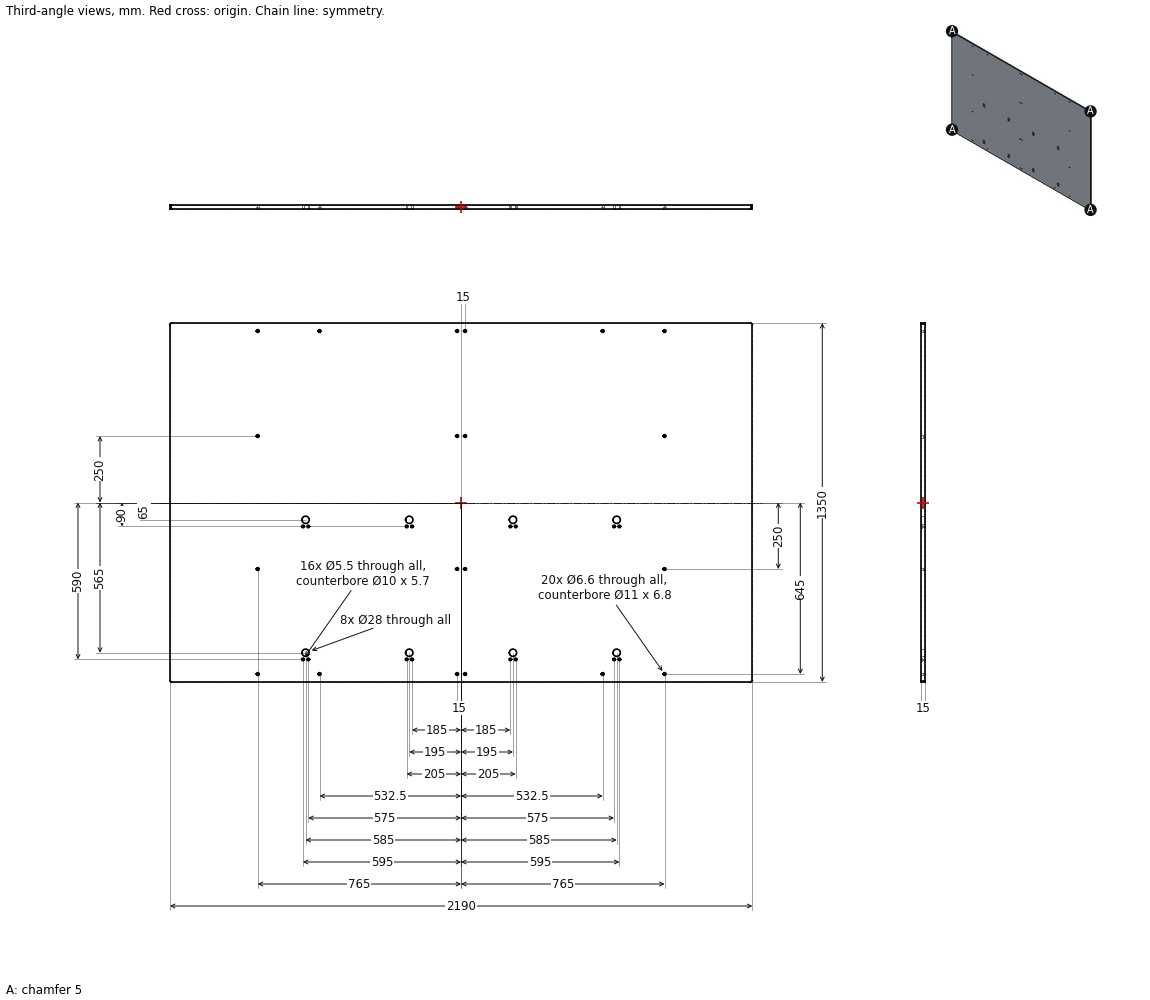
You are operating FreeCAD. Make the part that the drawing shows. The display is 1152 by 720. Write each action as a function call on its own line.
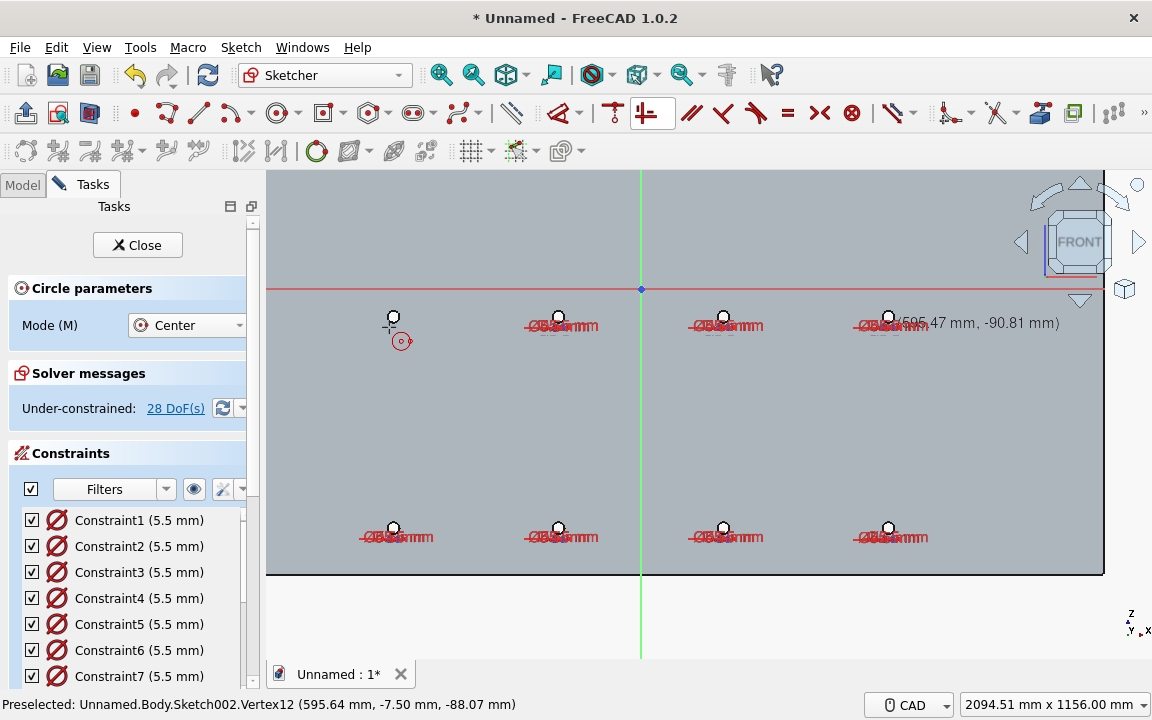
click(389, 327)
move(390, 326)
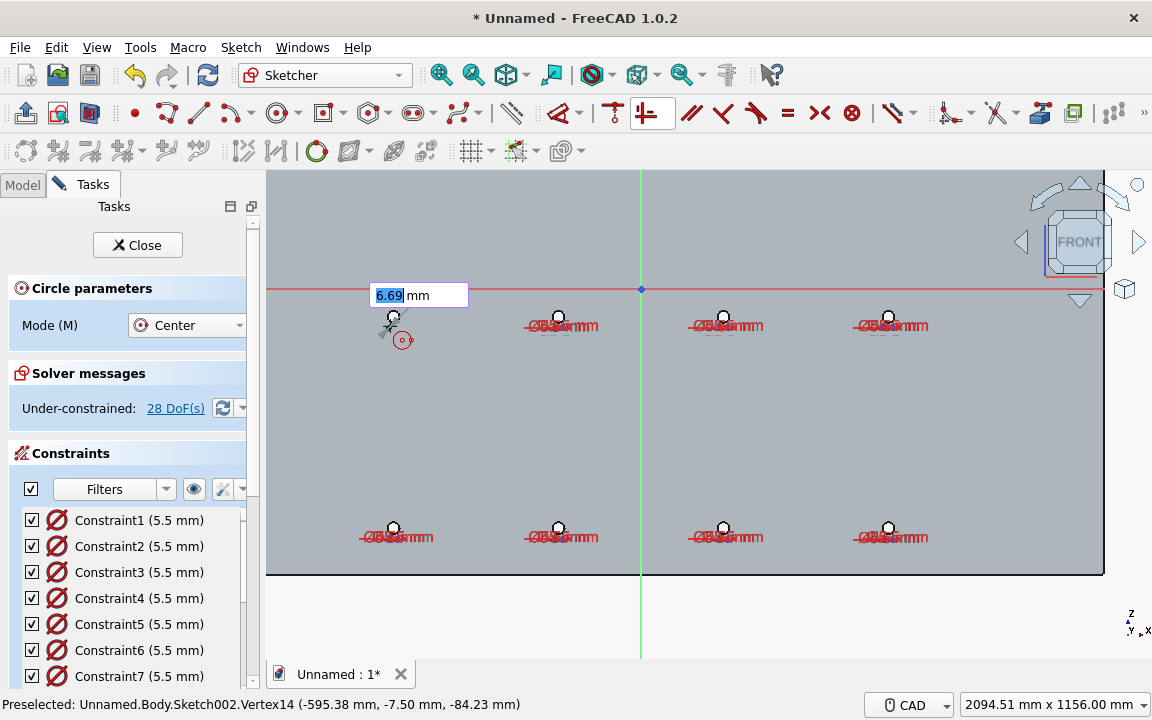
text(5.5)
key(Return)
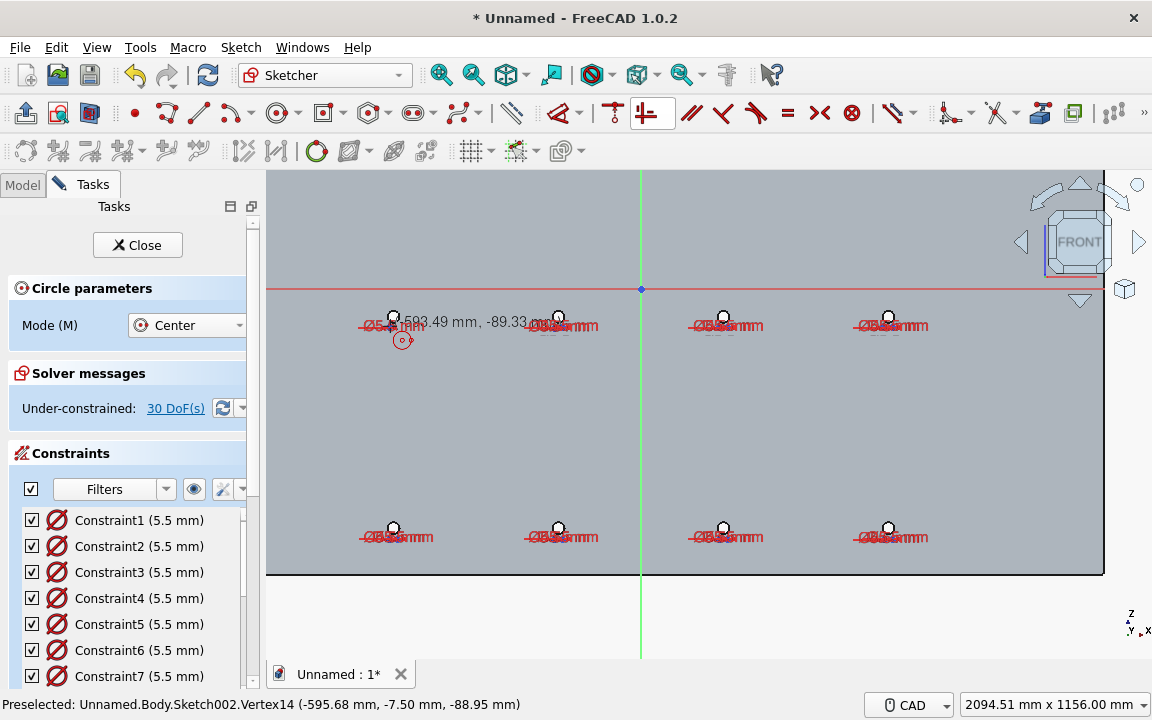
scroll(398, 327, up, 15)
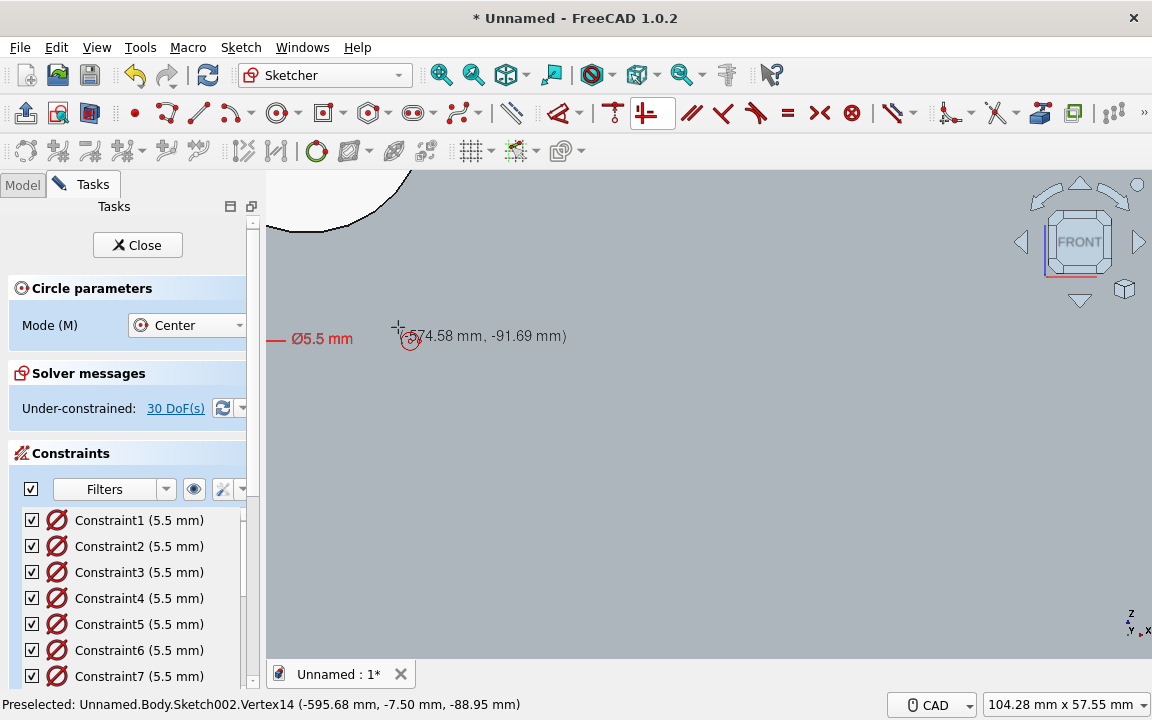
scroll(398, 327, down, 15)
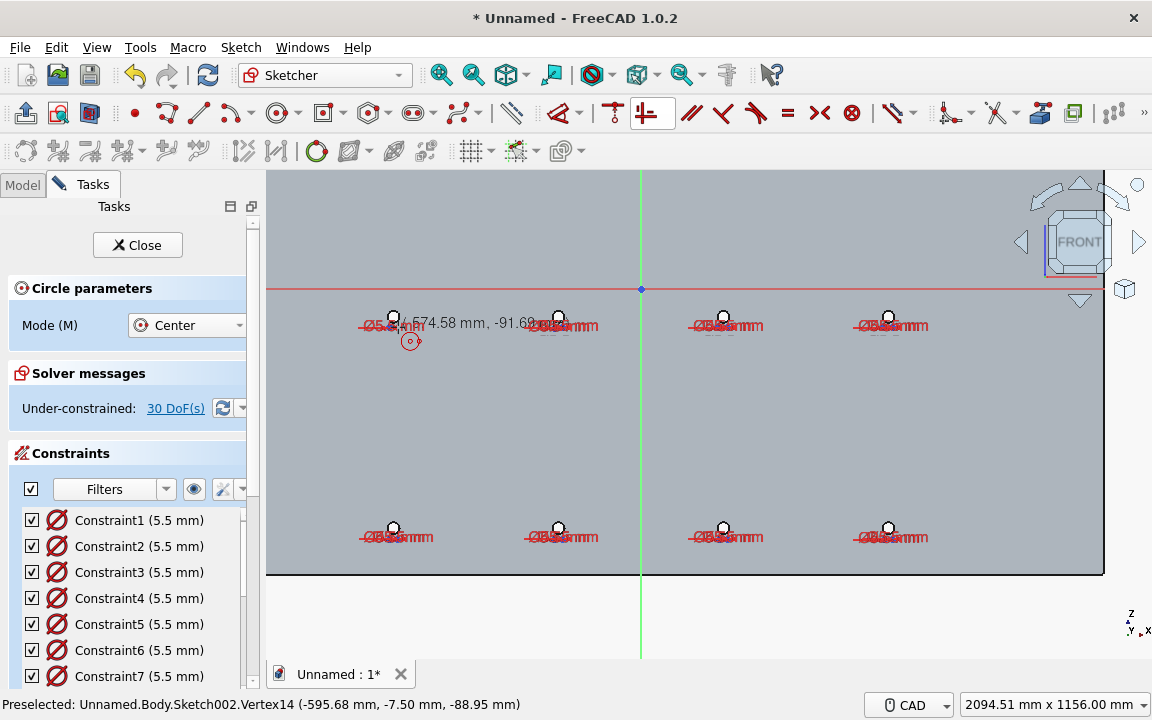
scroll(398, 327, up, 4)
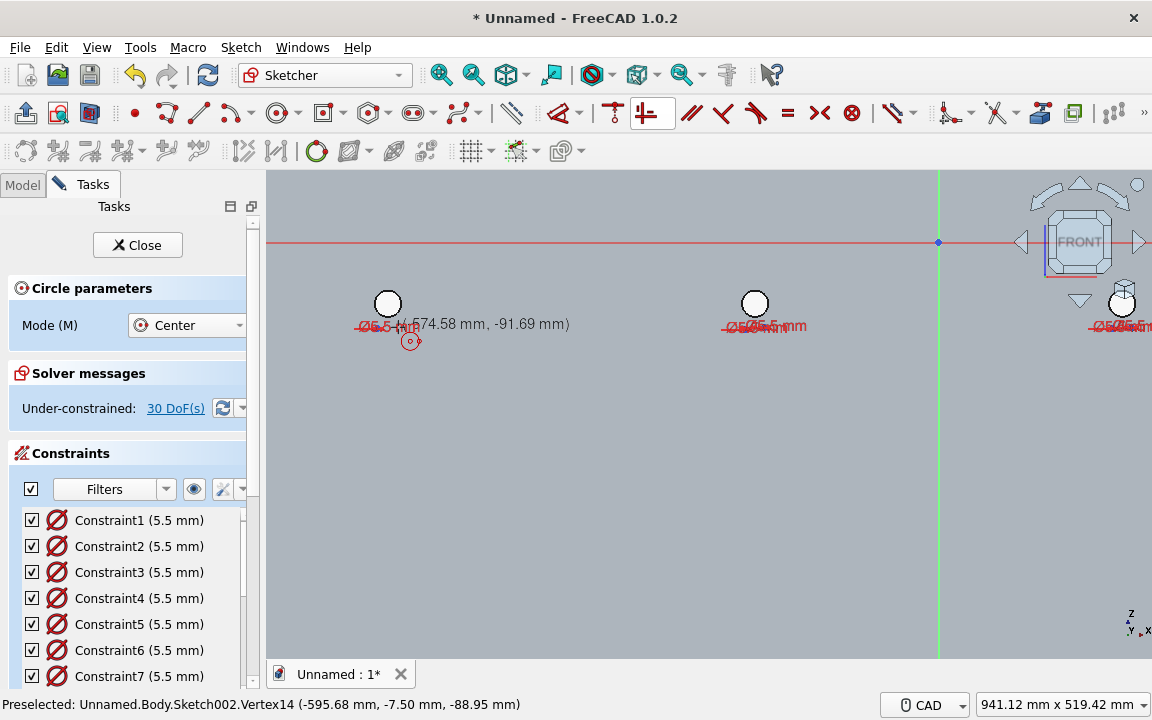
click(397, 327)
move(399, 325)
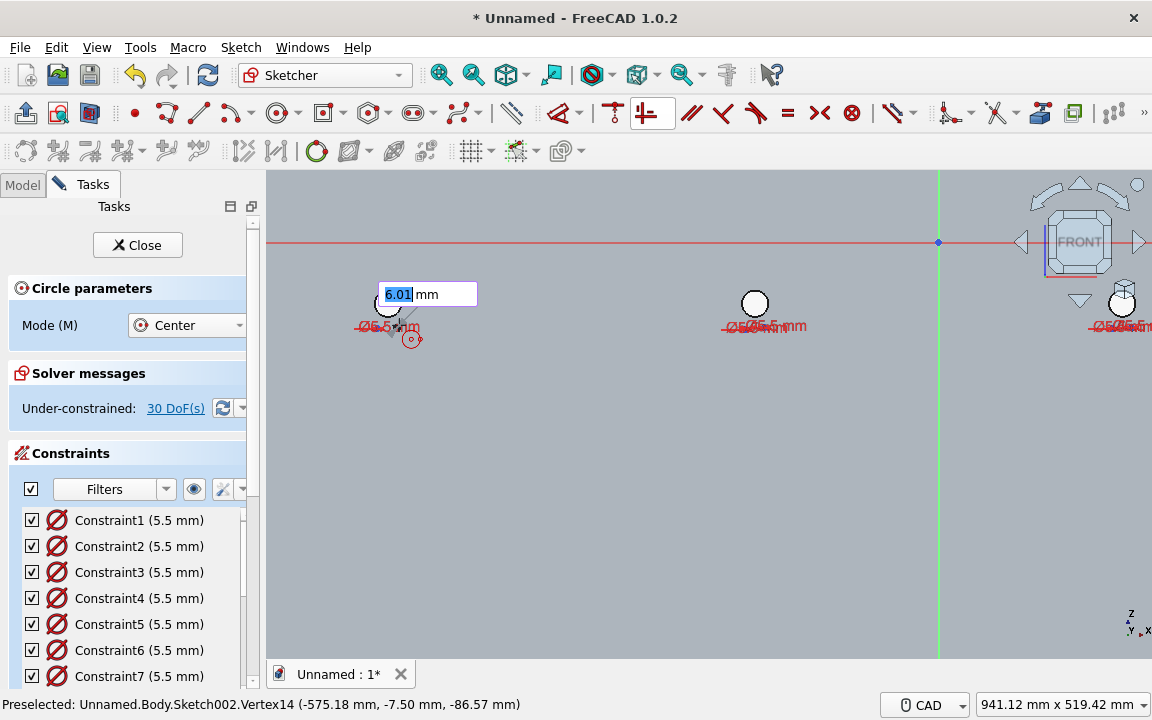
text(5.5)
key(Return)
key(Escape)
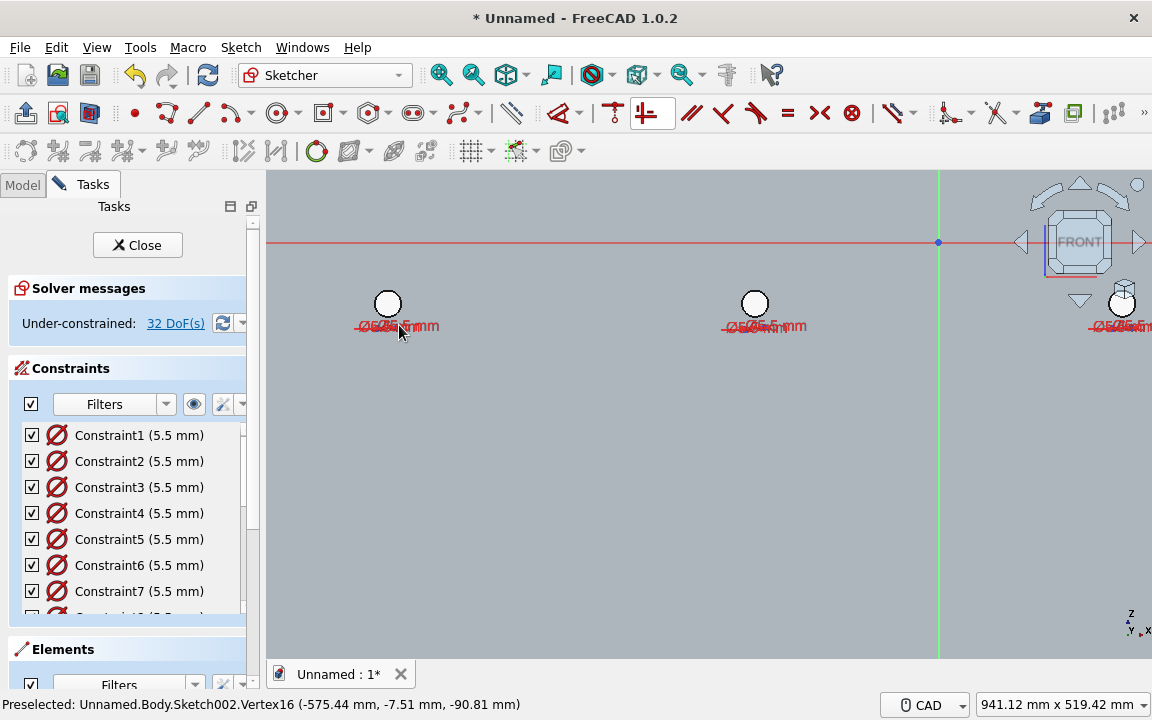
scroll(397, 327, down, 4)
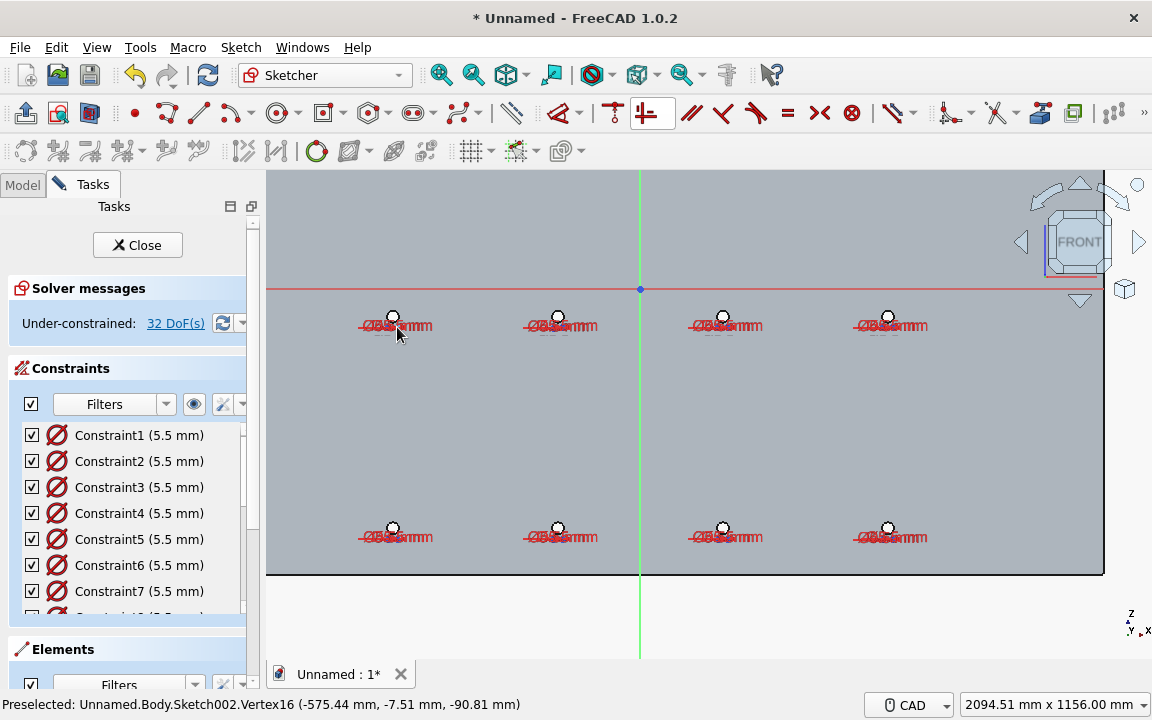
scroll(389, 539, up, 2)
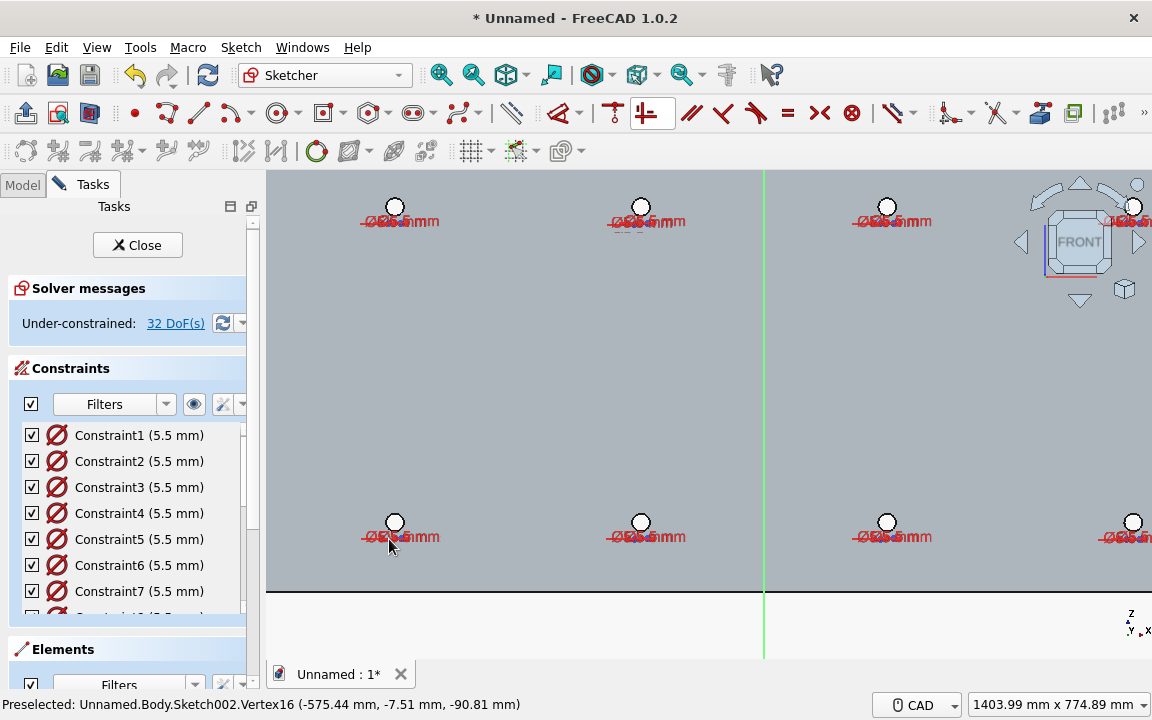
click(389, 539)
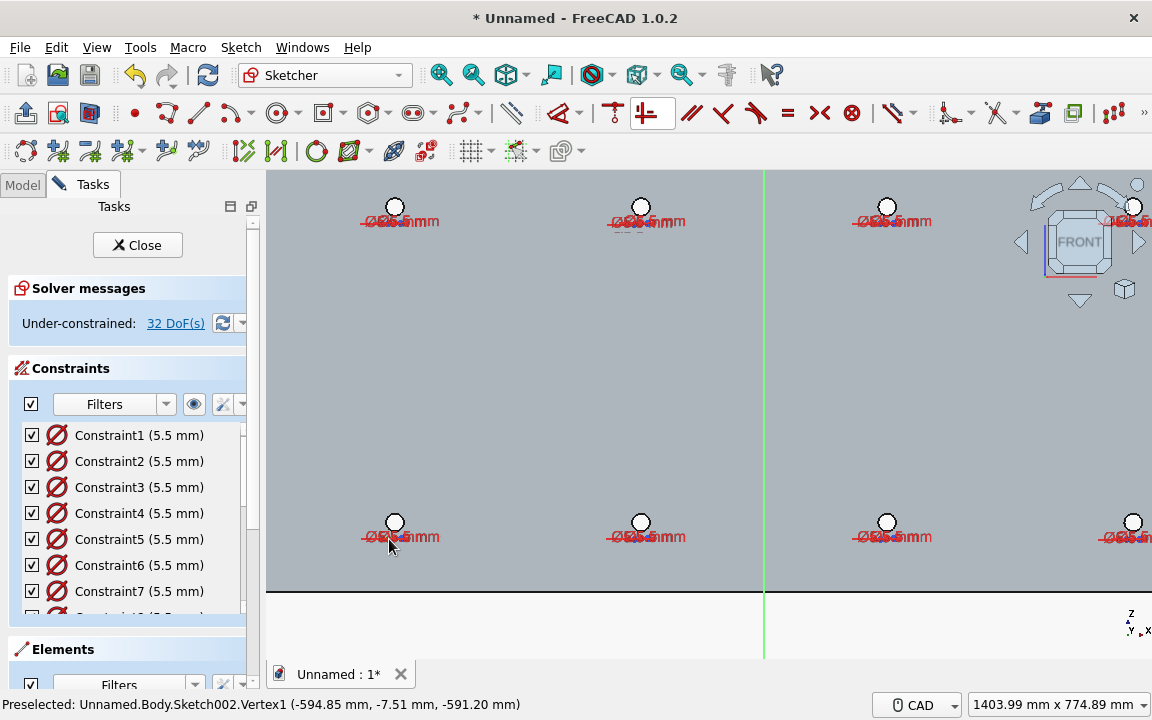
click(401, 539)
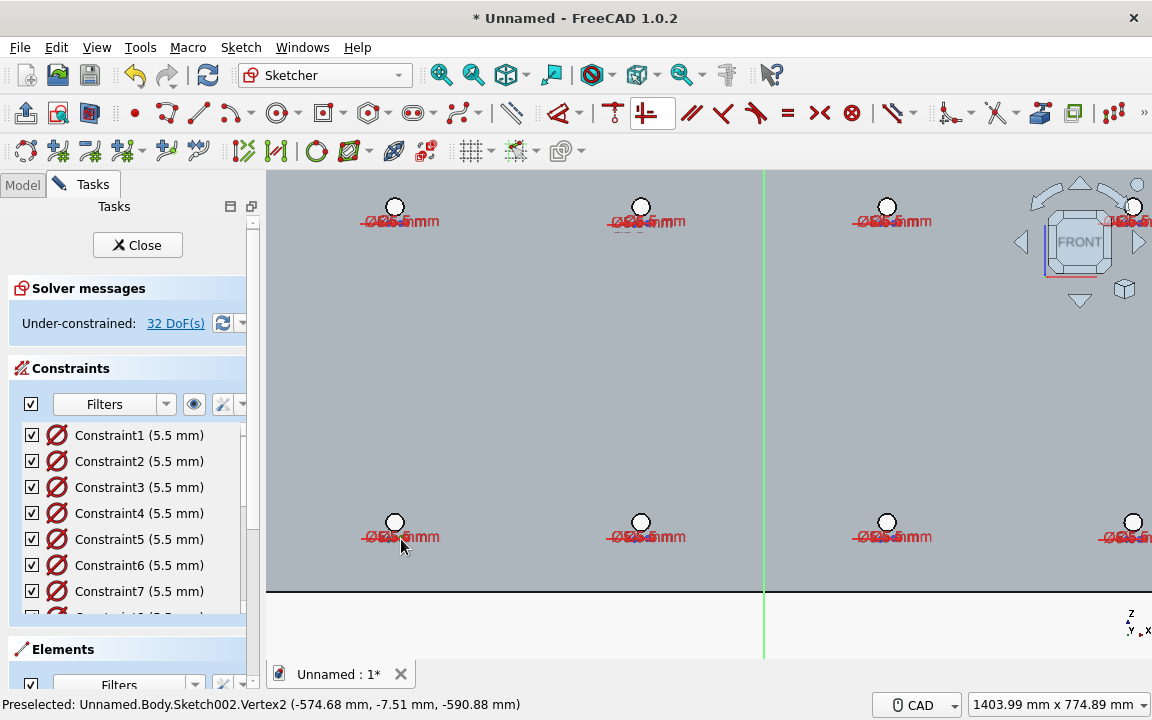
key(h)